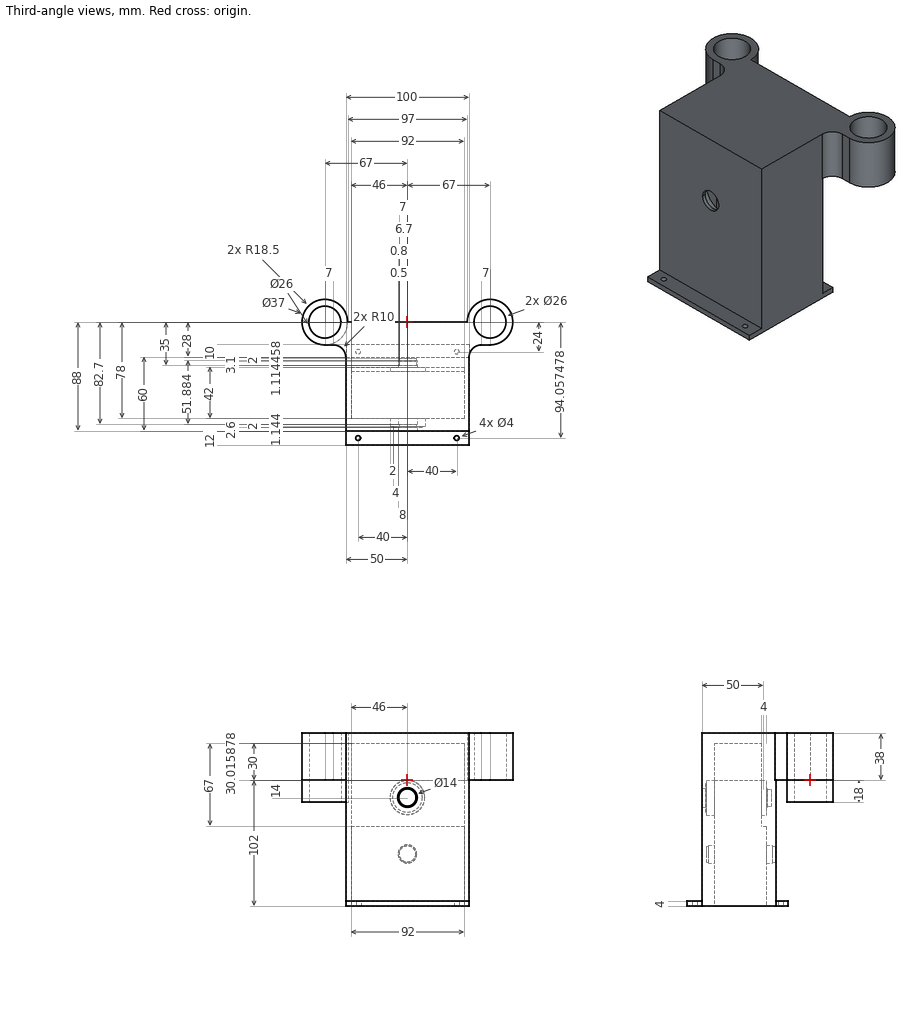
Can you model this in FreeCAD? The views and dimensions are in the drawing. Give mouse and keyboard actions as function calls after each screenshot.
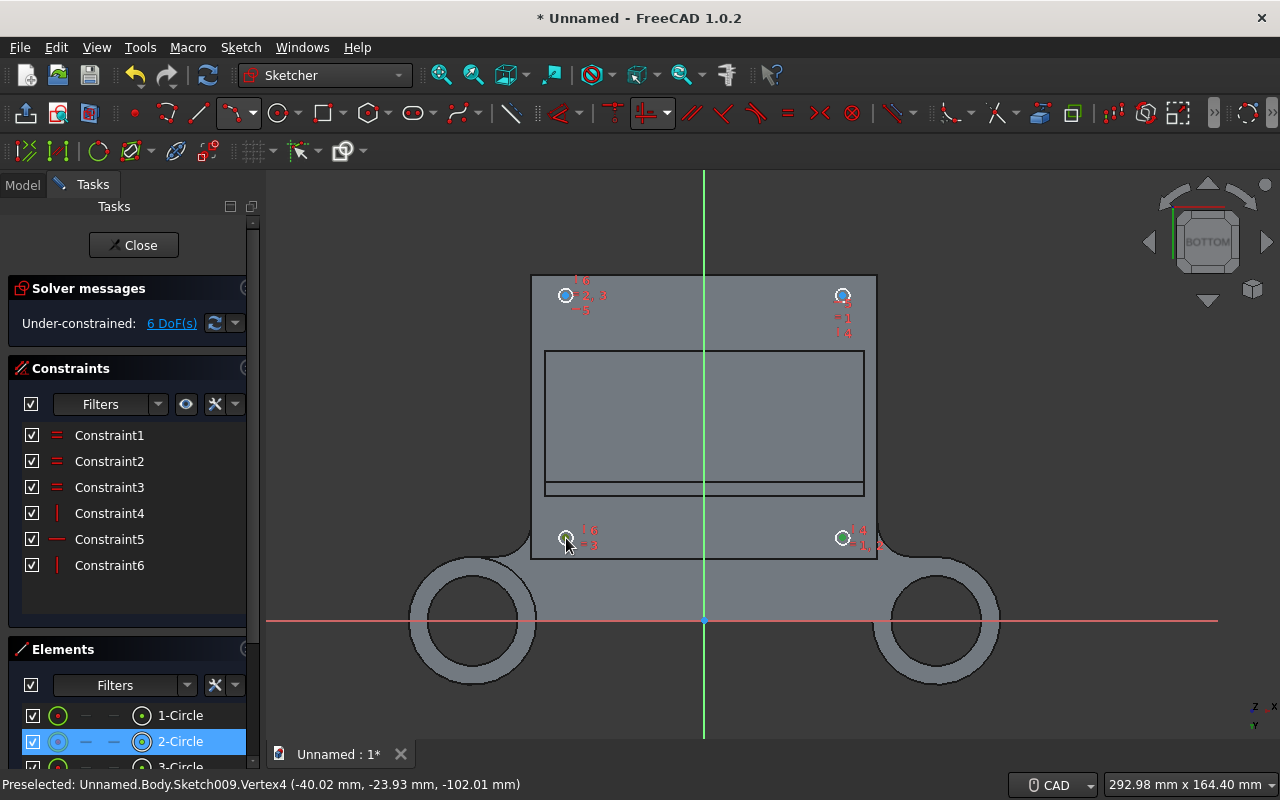
key(h)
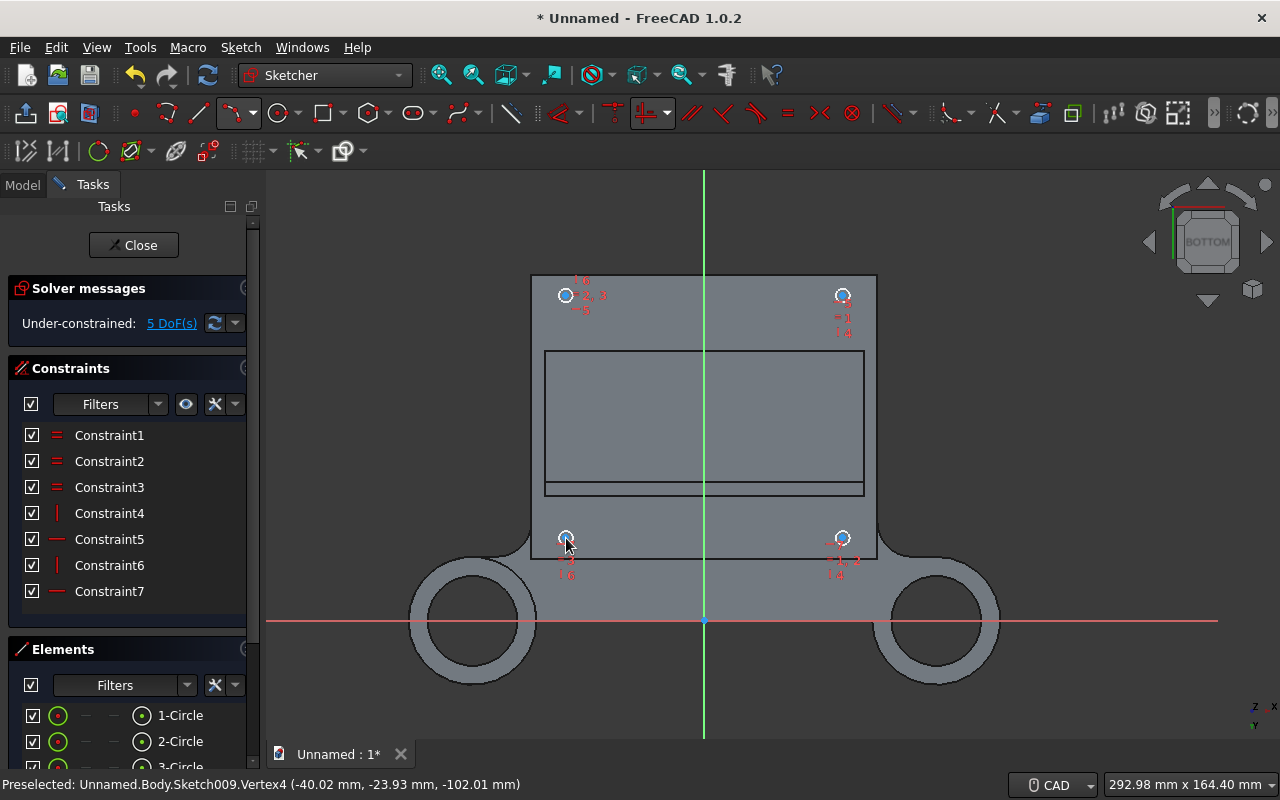
click(558, 114)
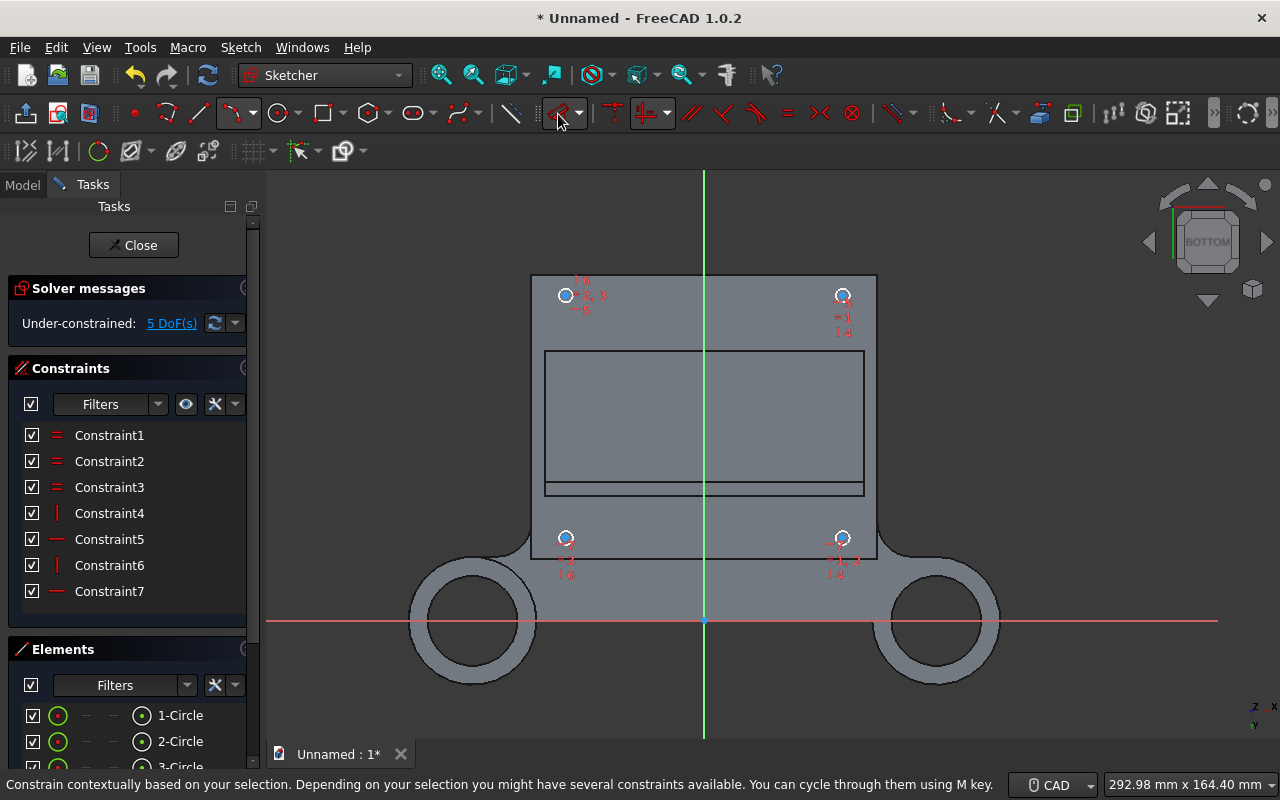
scroll(836, 295, up, 6)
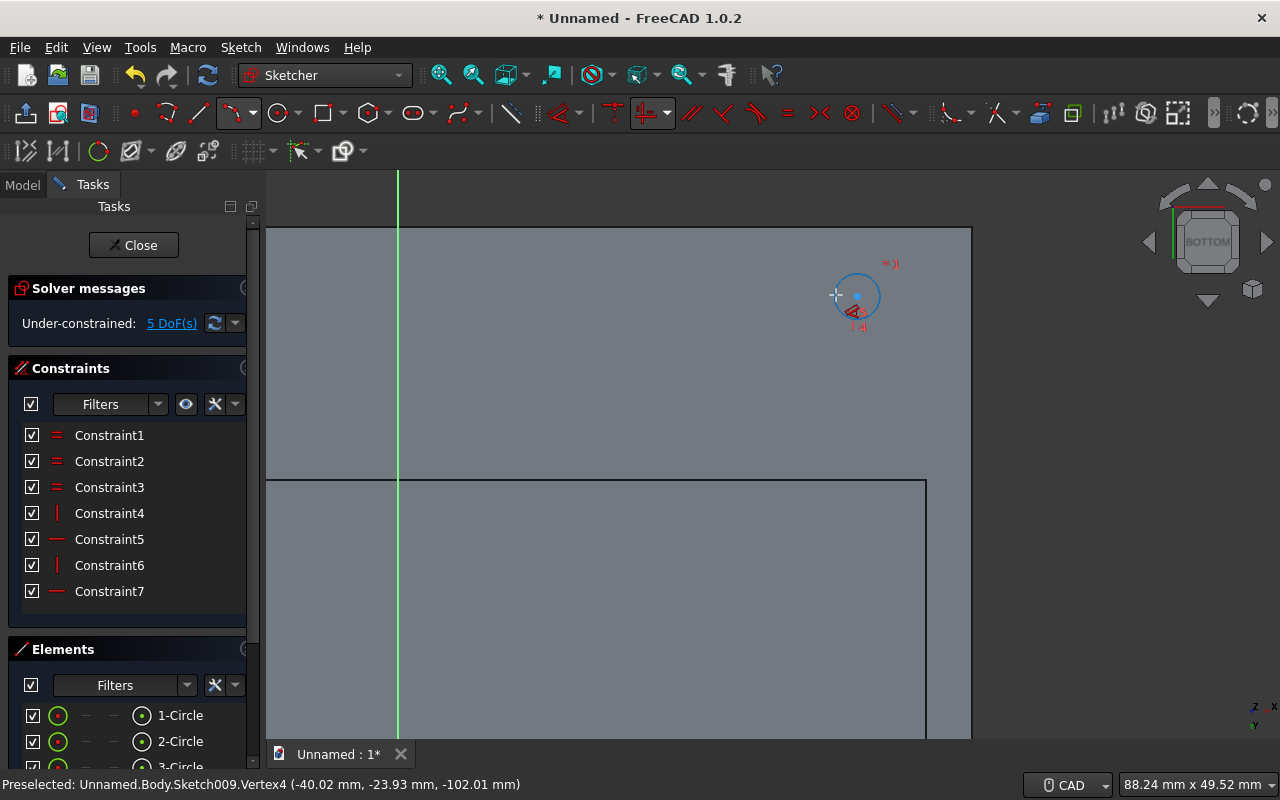
click(835, 296)
click(803, 295)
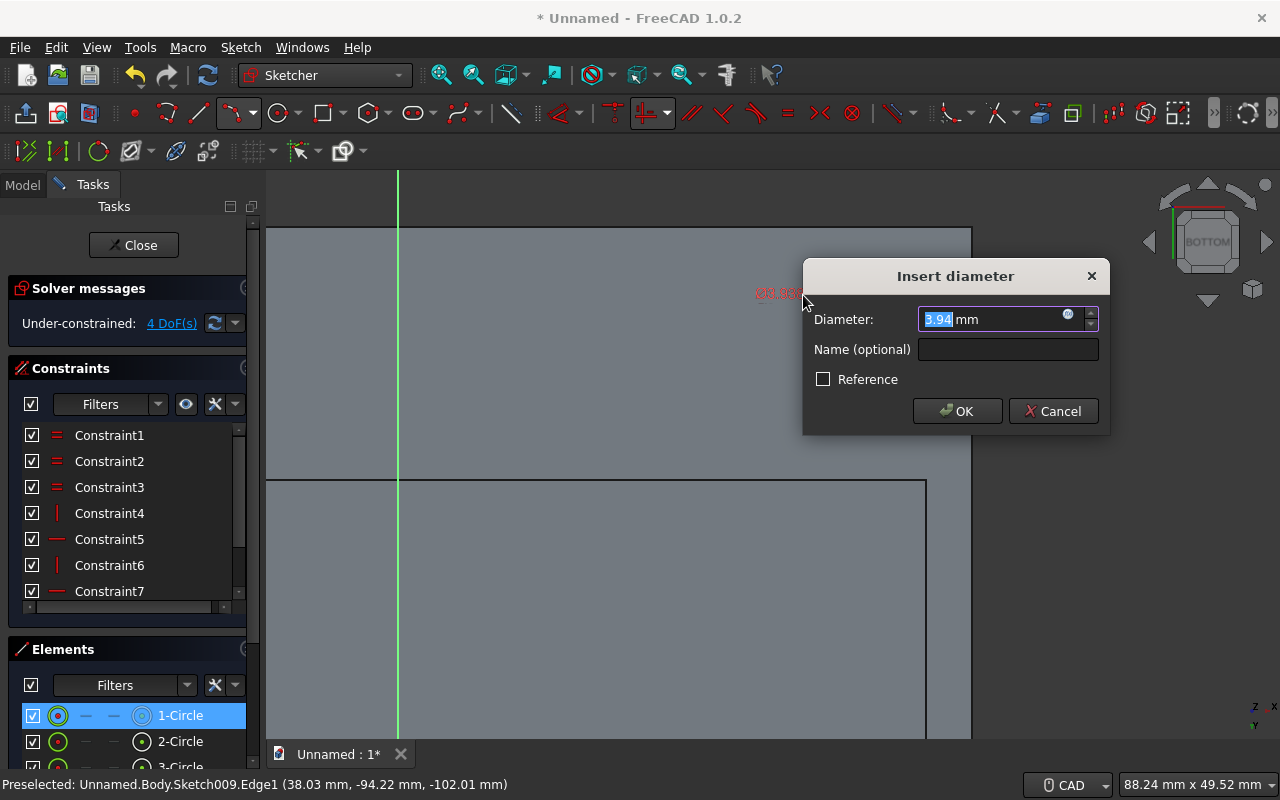
text(4)
key(Return)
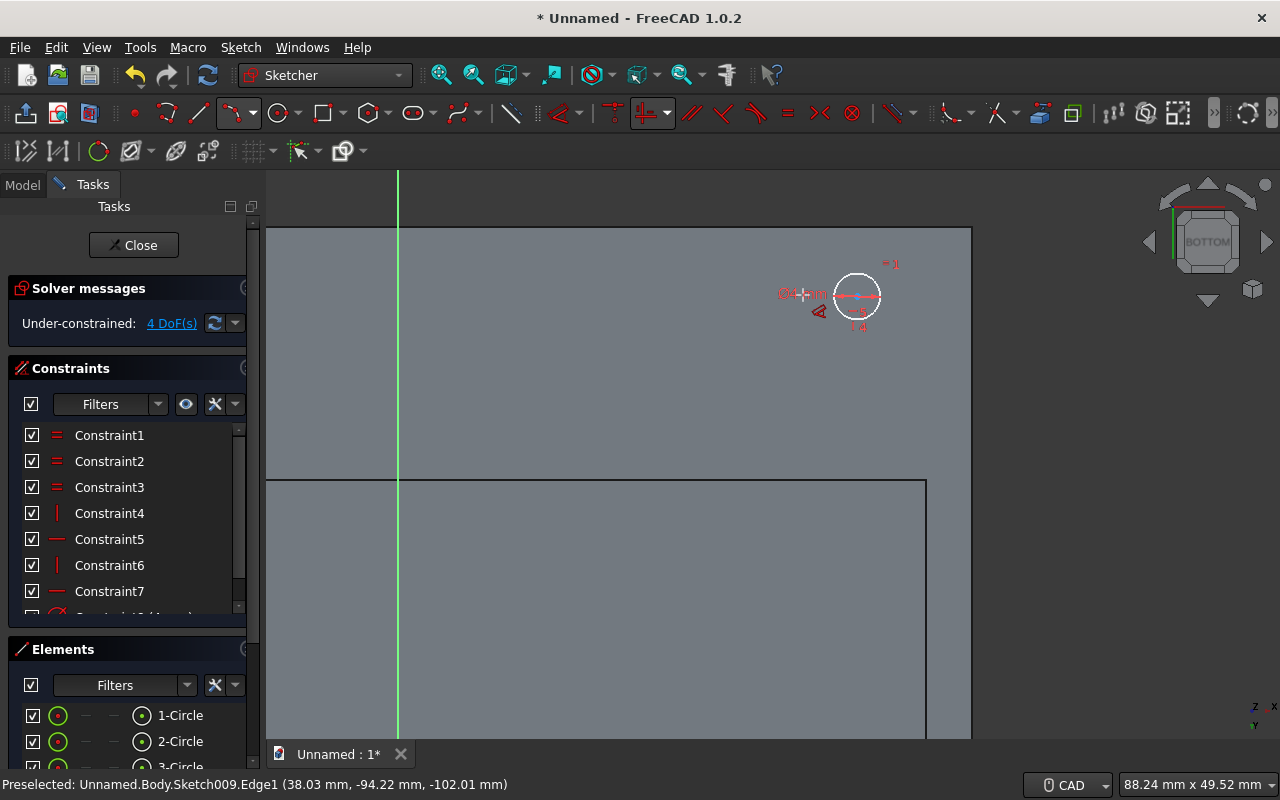
click(857, 296)
click(628, 262)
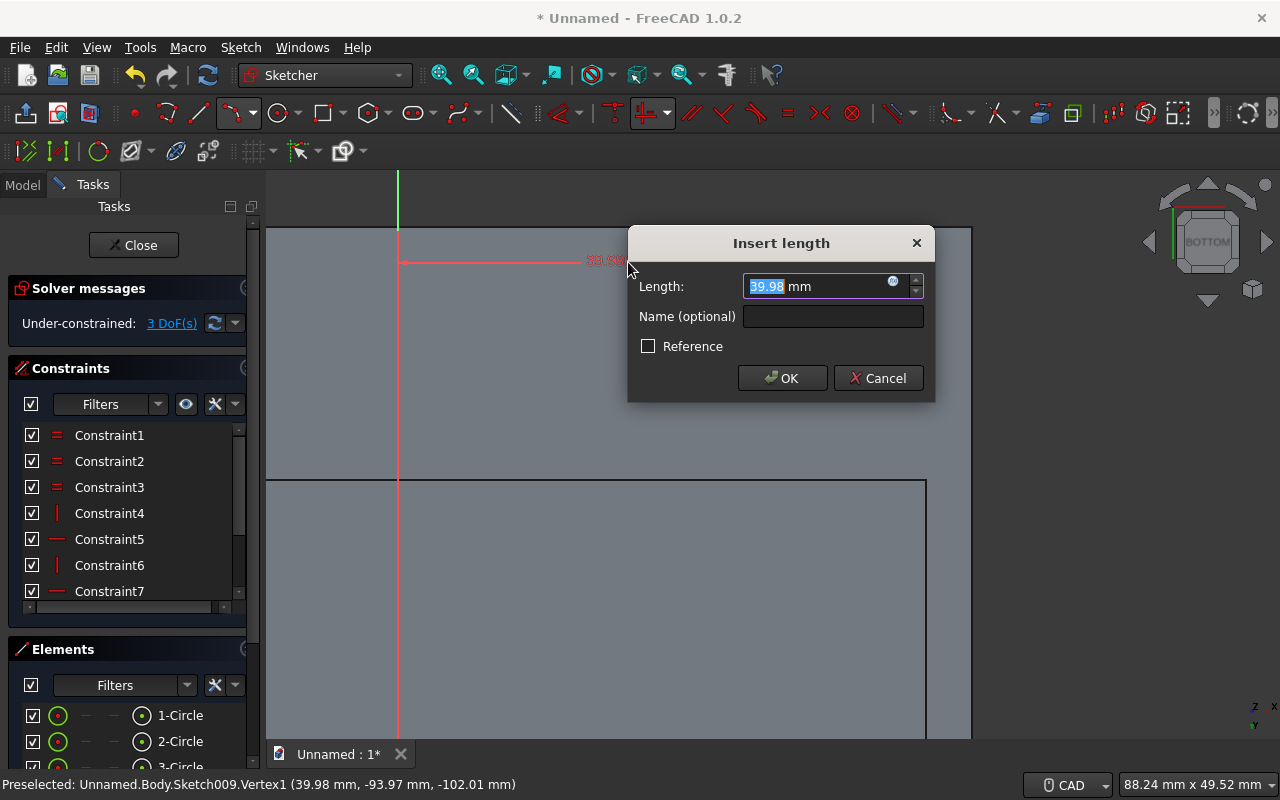
text(40)
key(Return)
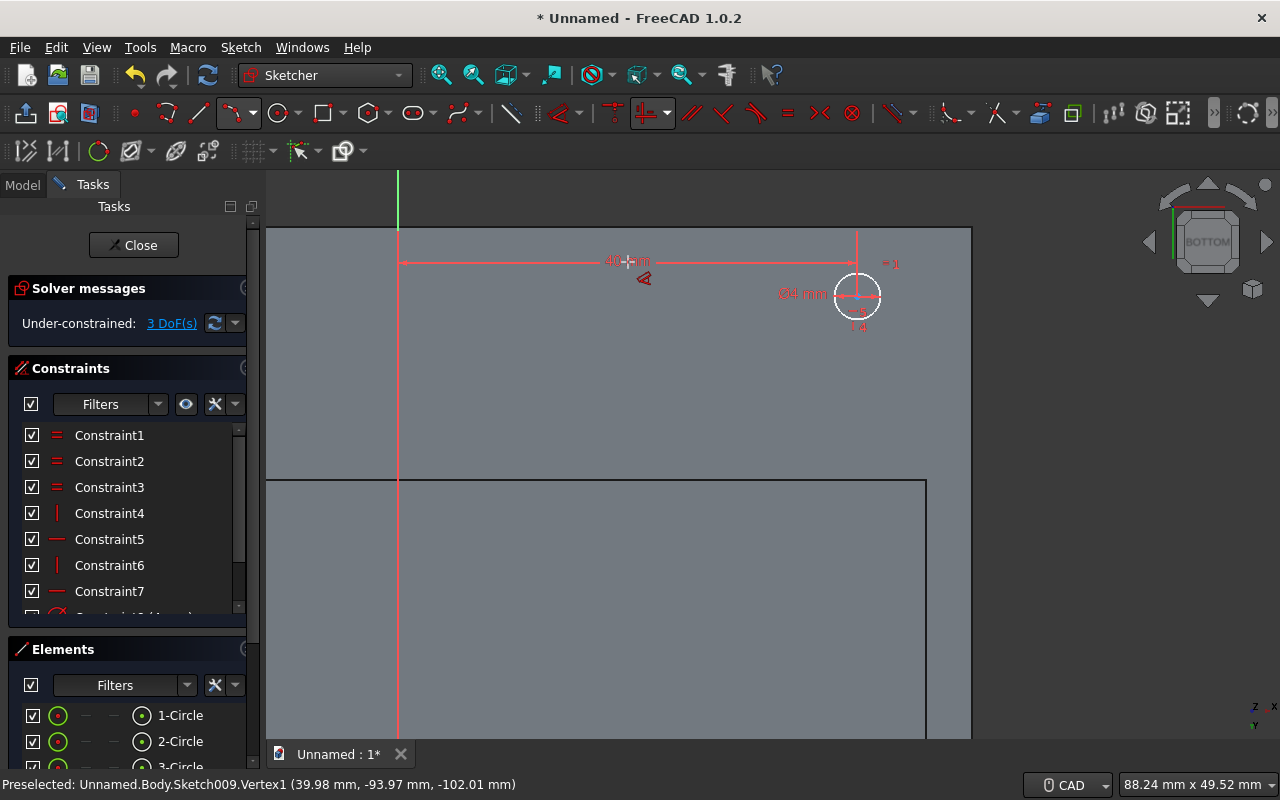
scroll(837, 295, down, 6)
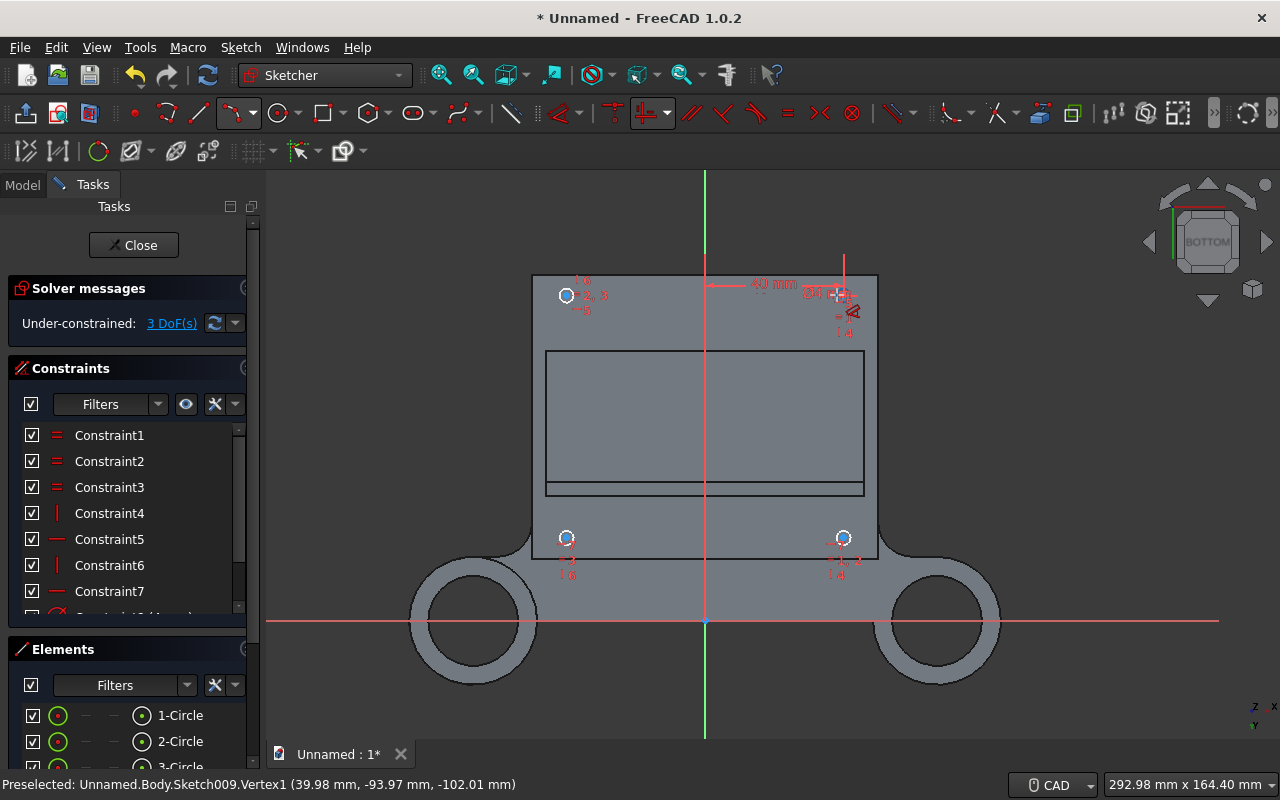
click(844, 538)
click(878, 579)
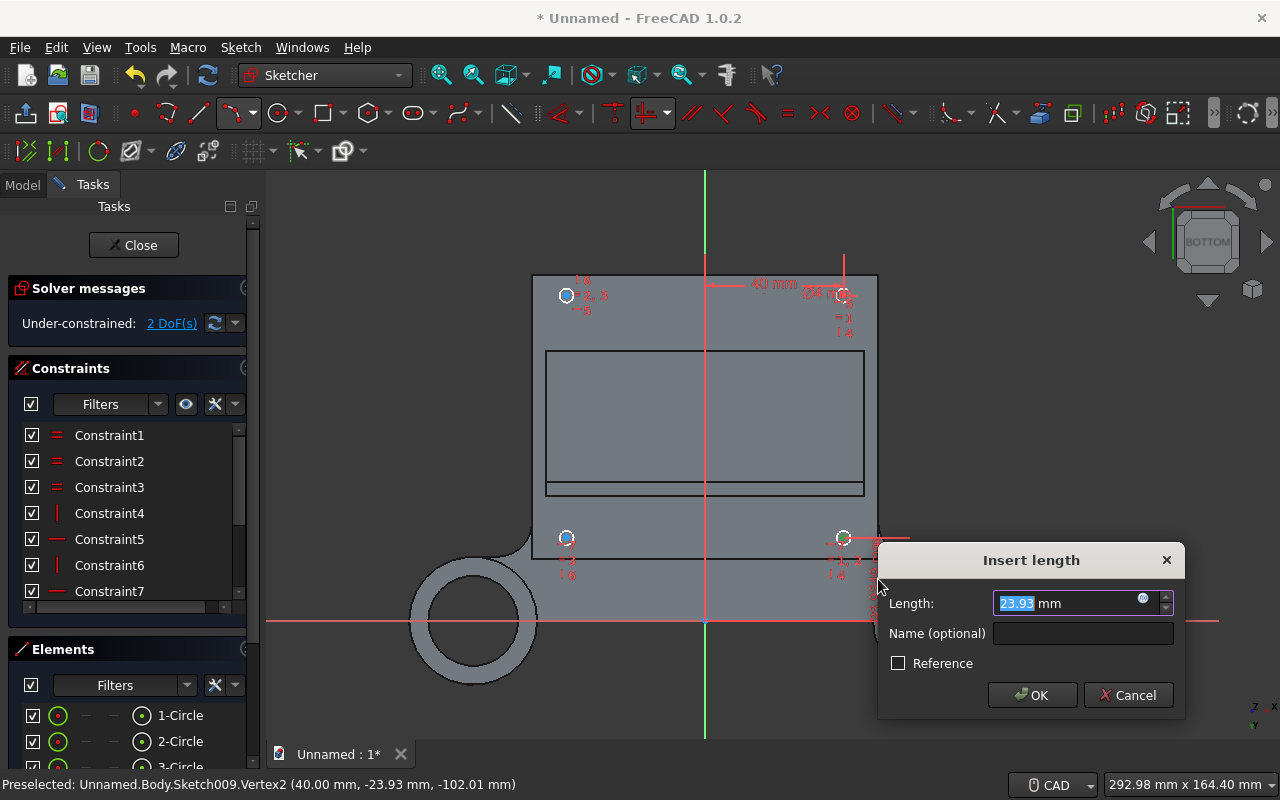
text(24)
key(Return)